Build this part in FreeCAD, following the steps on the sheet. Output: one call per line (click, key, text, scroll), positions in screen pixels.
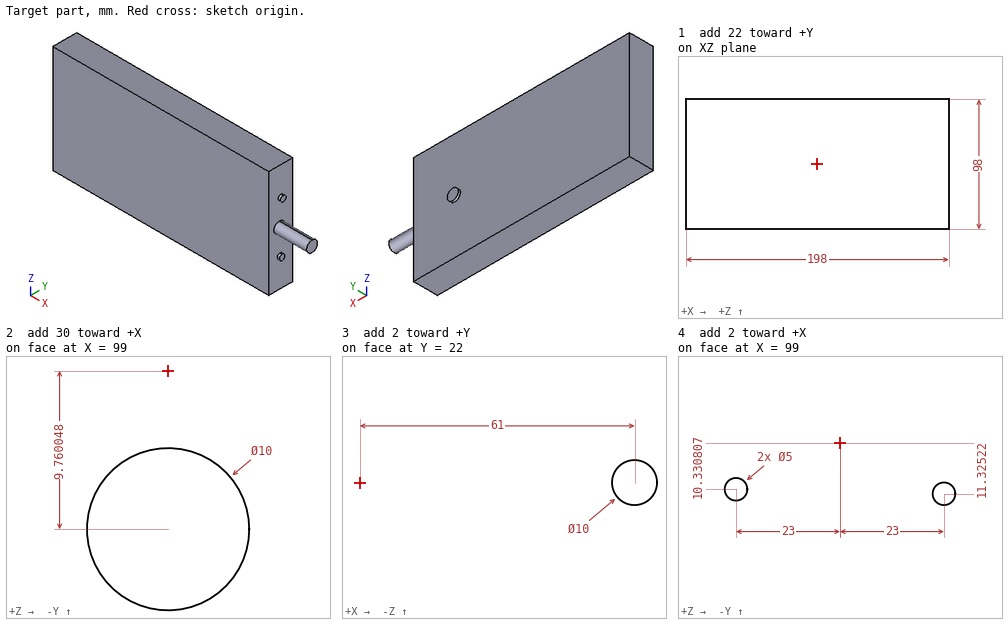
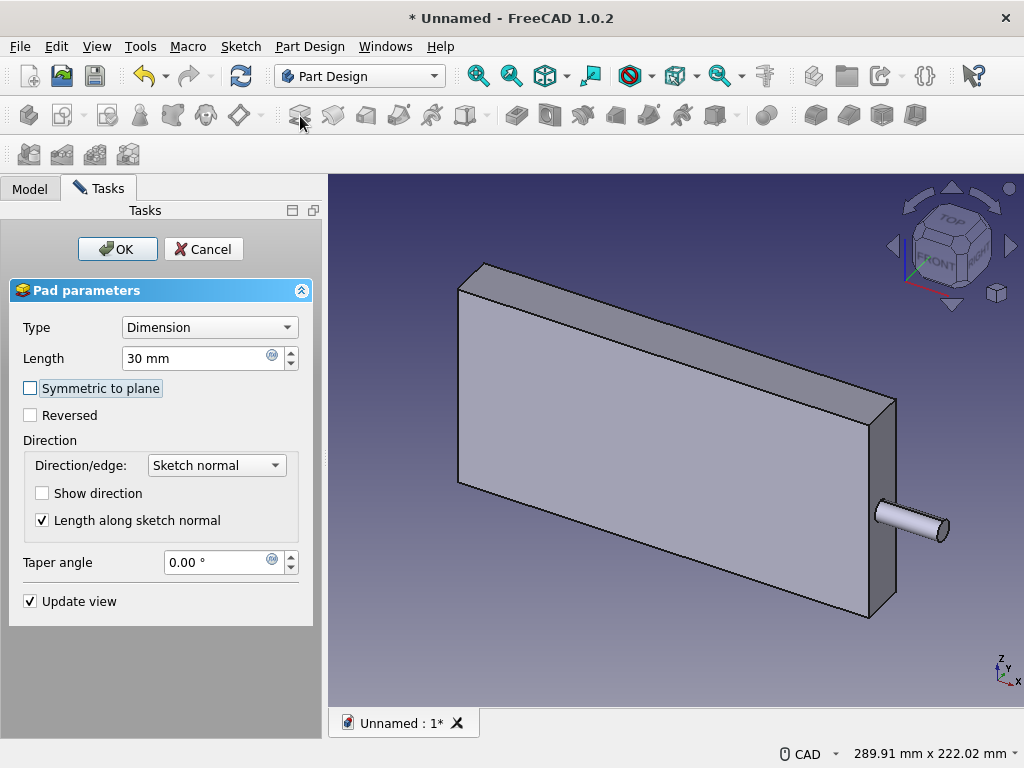
click(118, 249)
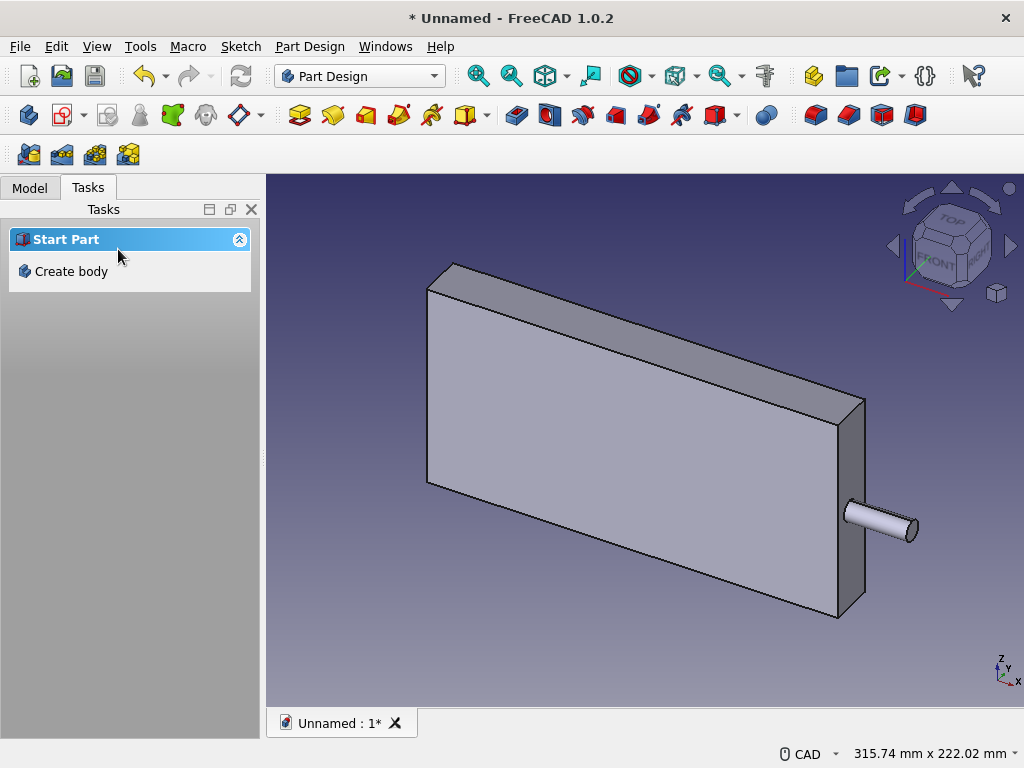
key(4)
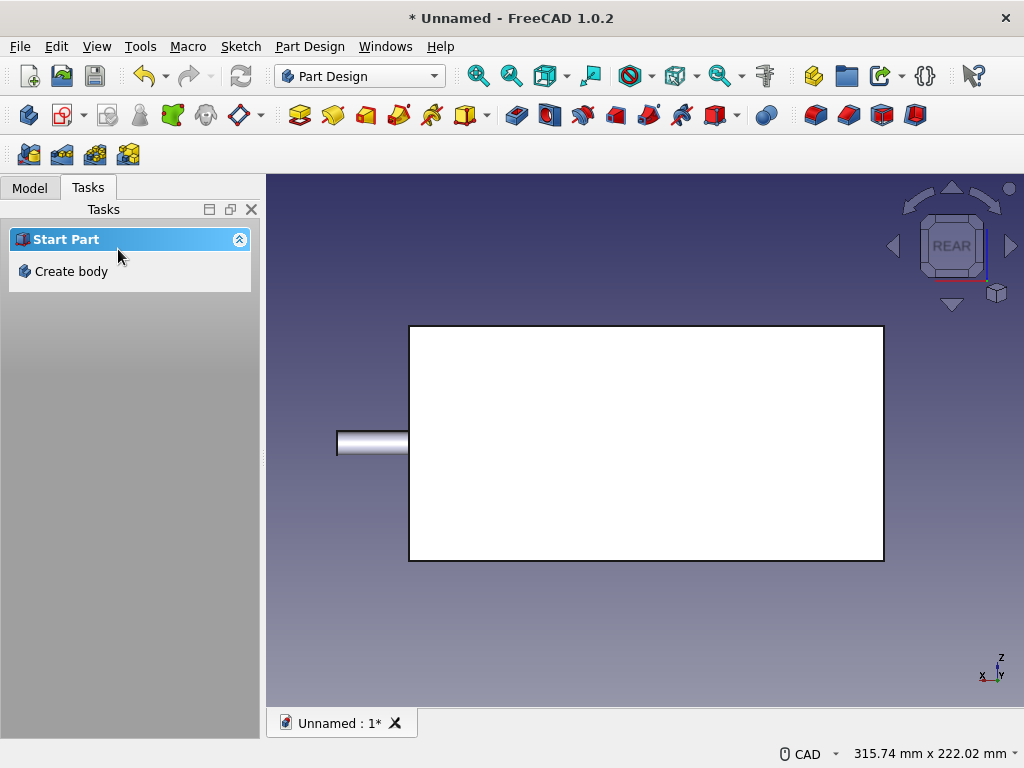
click(578, 442)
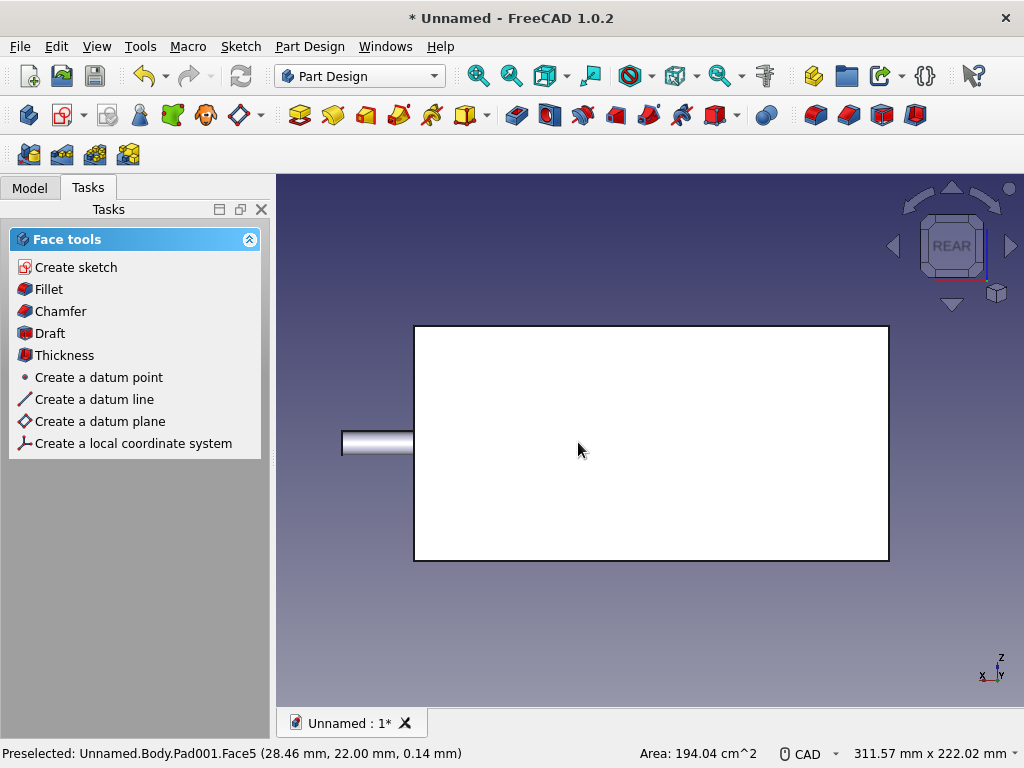
click(62, 116)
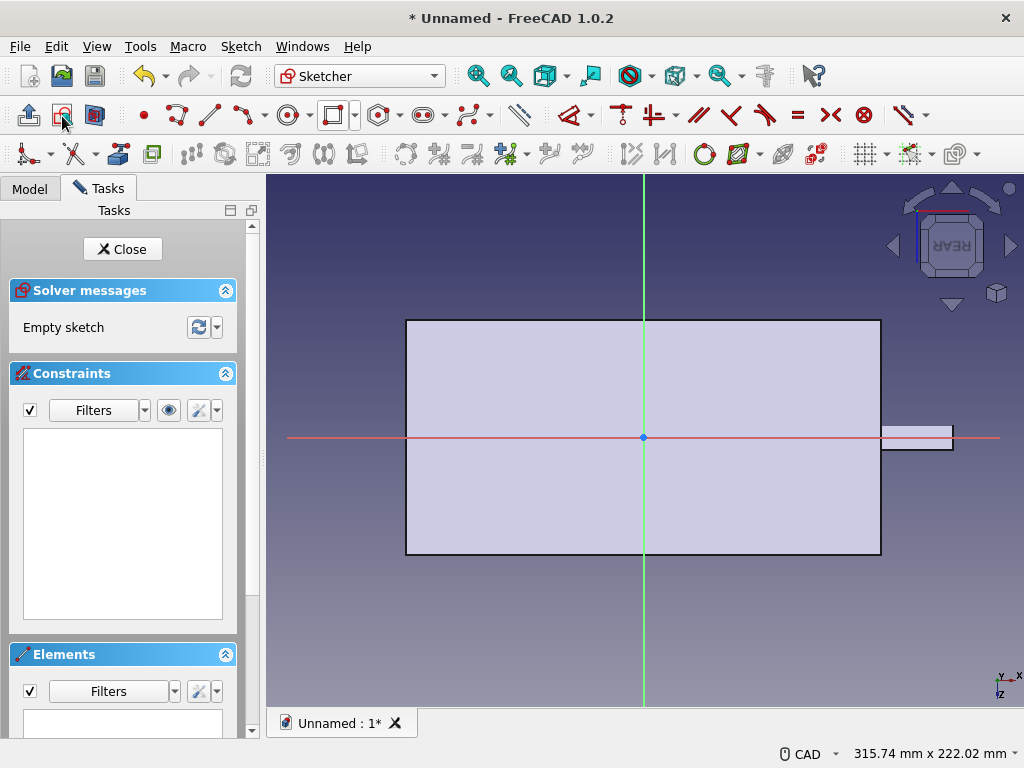
scroll(807, 437, up, 13)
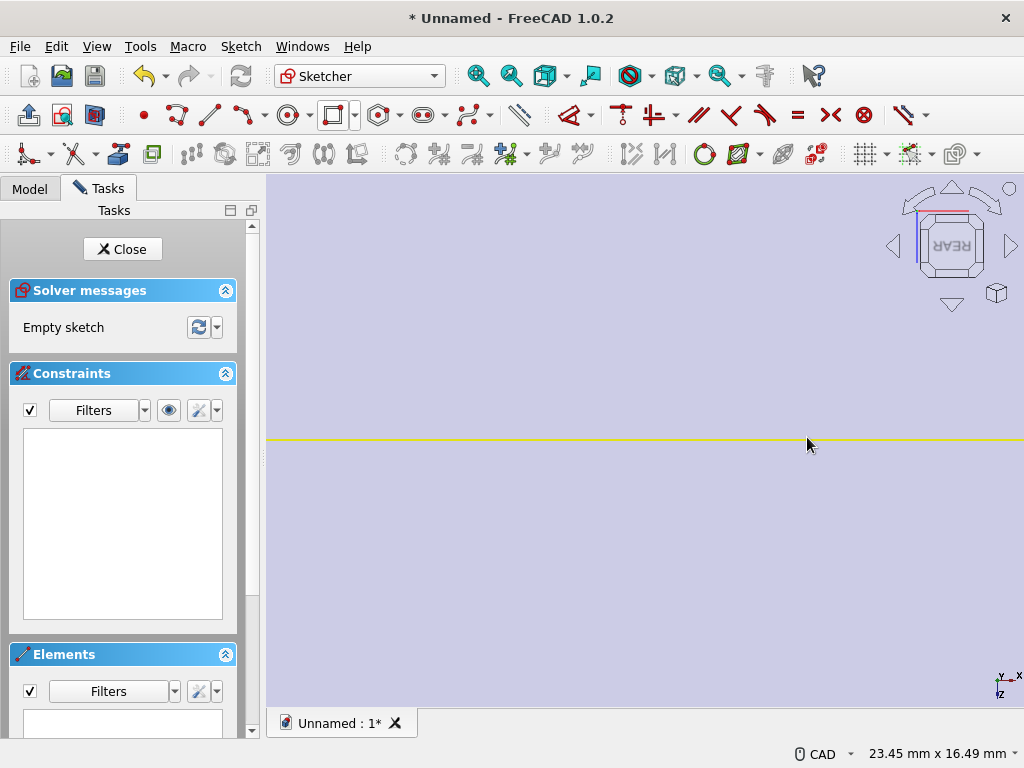
key(g)
key(c)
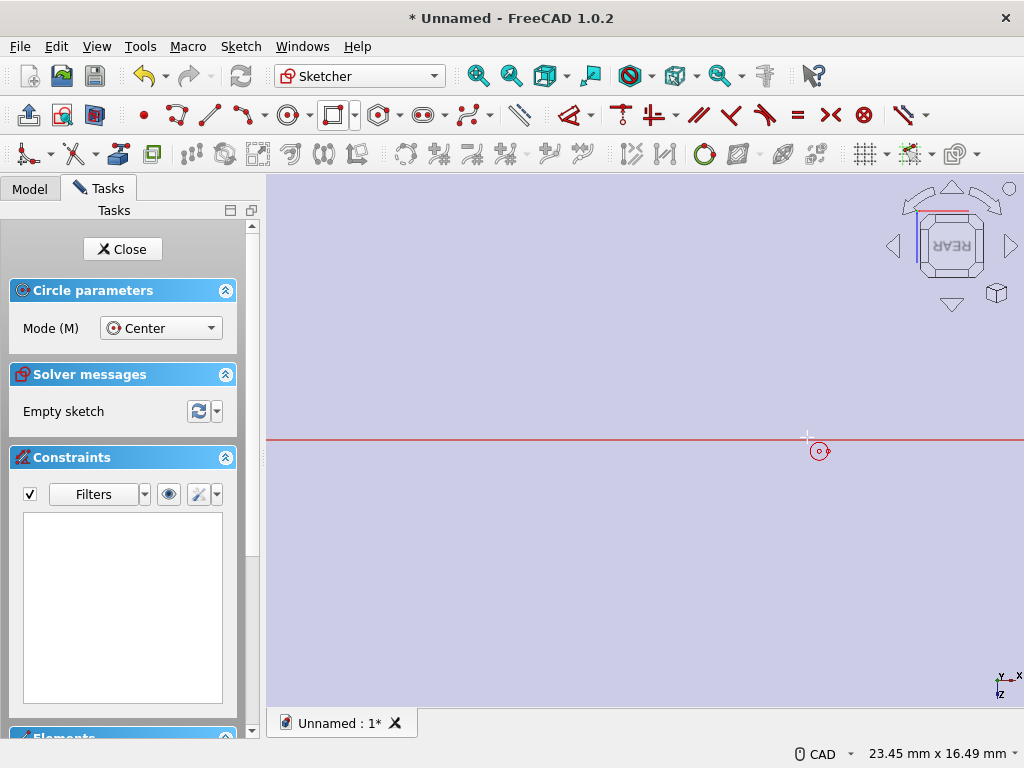
click(571, 440)
move(685, 325)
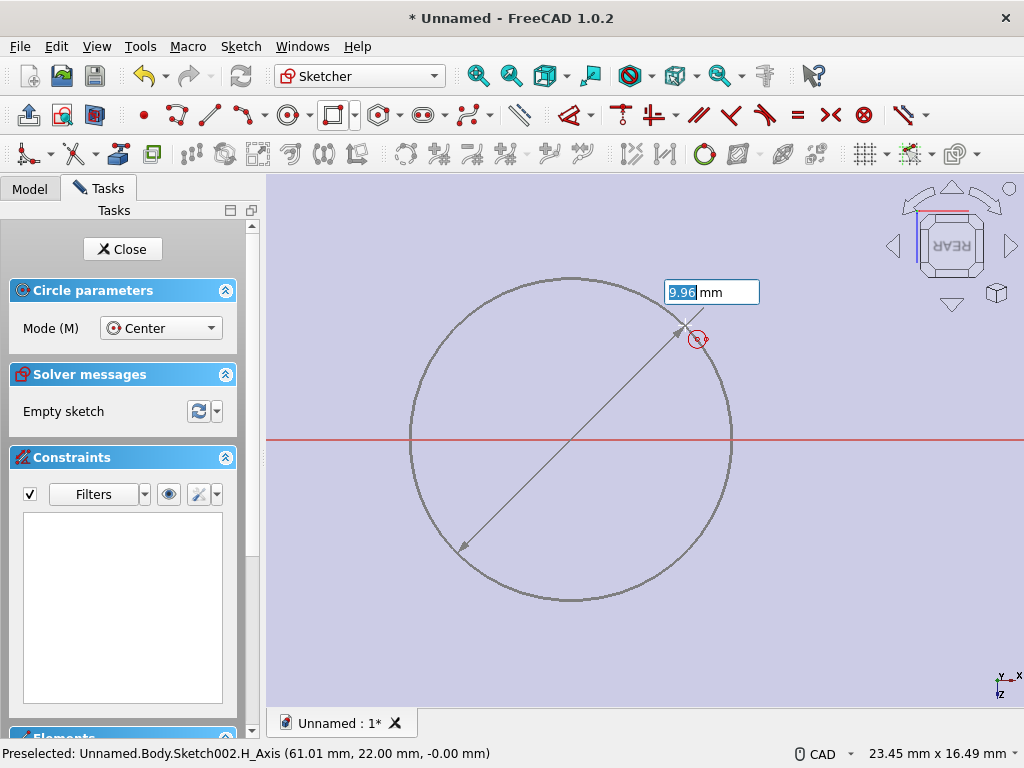
text(10)
key(Return)
key(Escape)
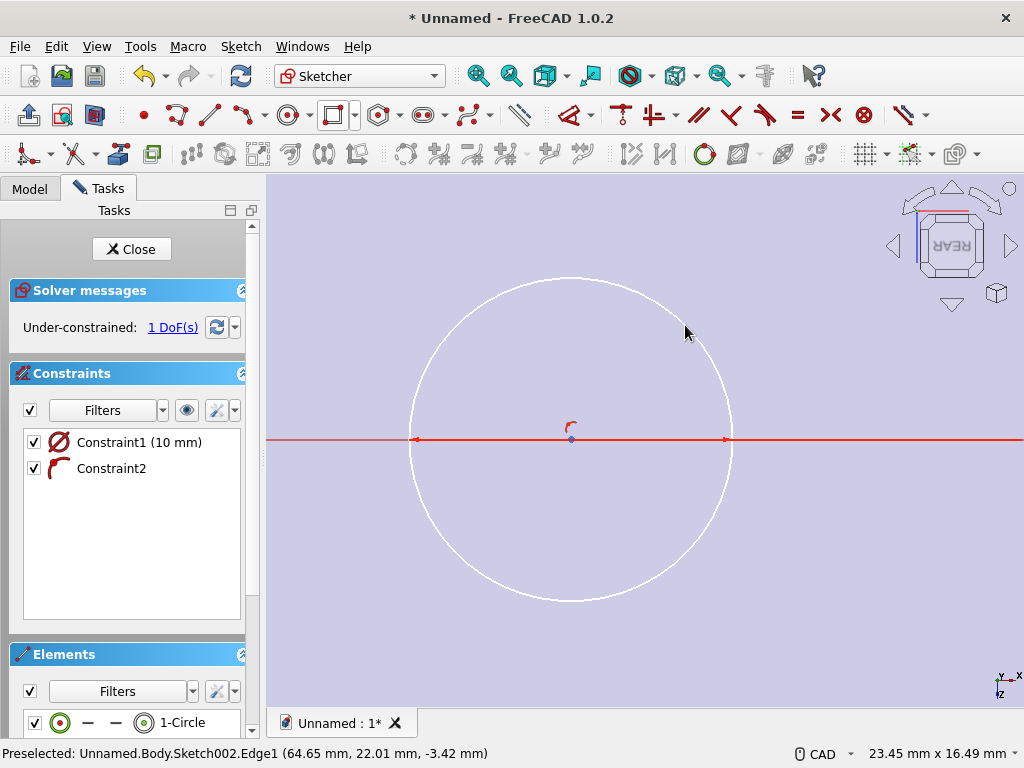
key(d)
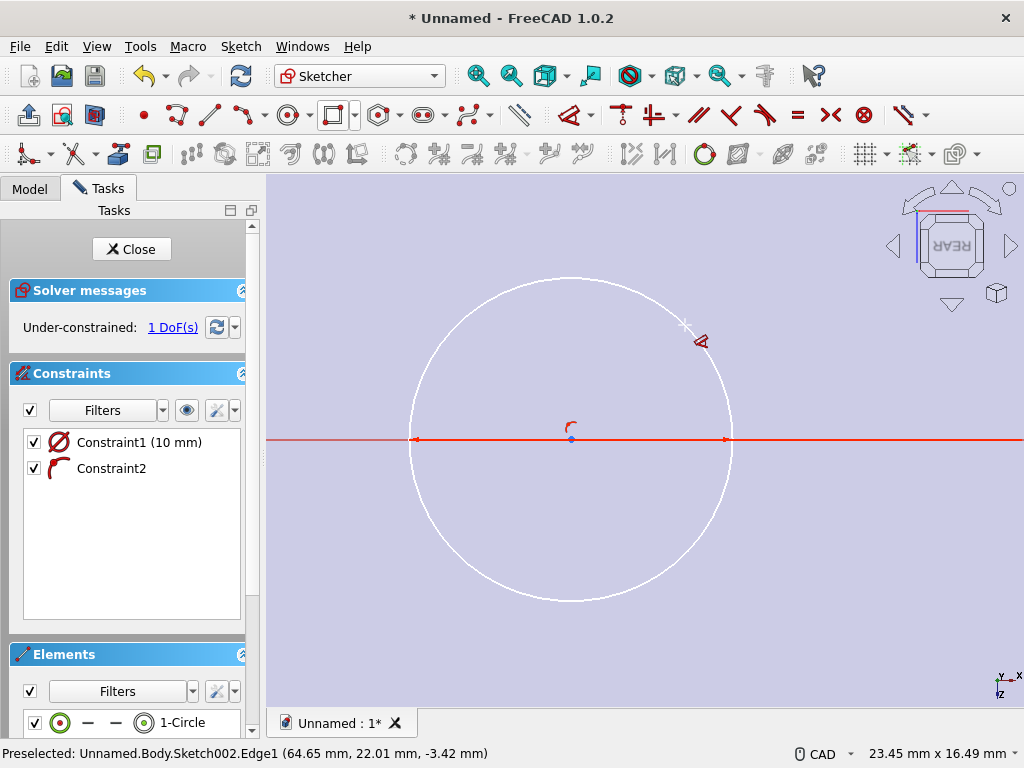
click(571, 440)
click(433, 474)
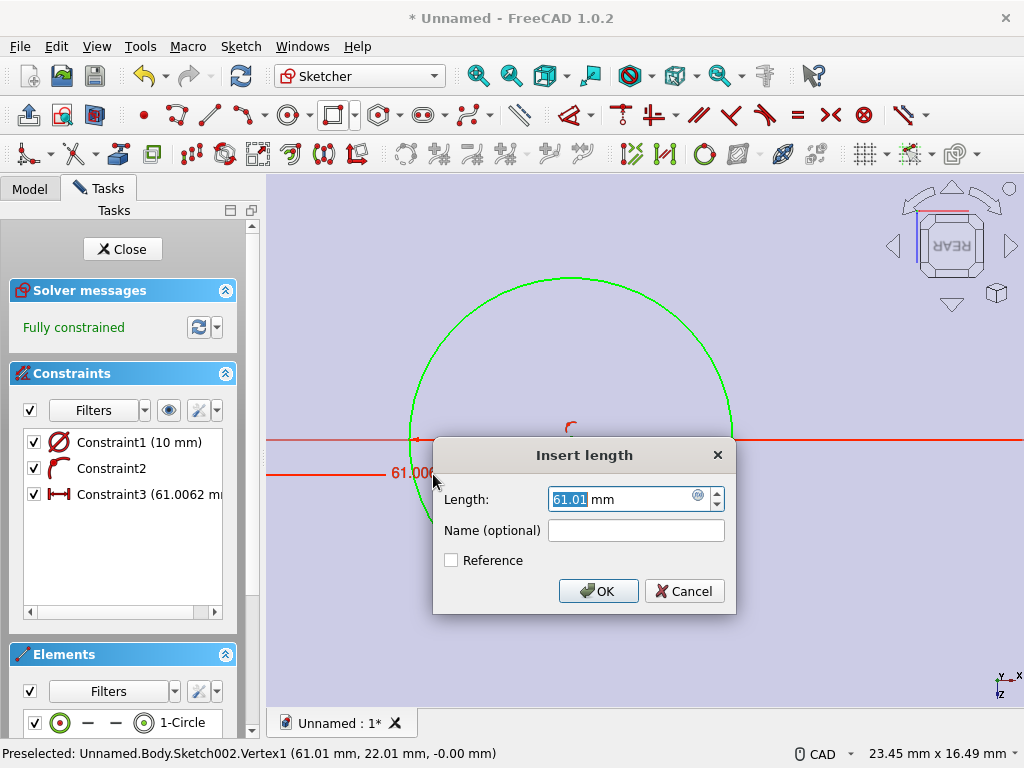
text(61)
key(Return)
key(Escape)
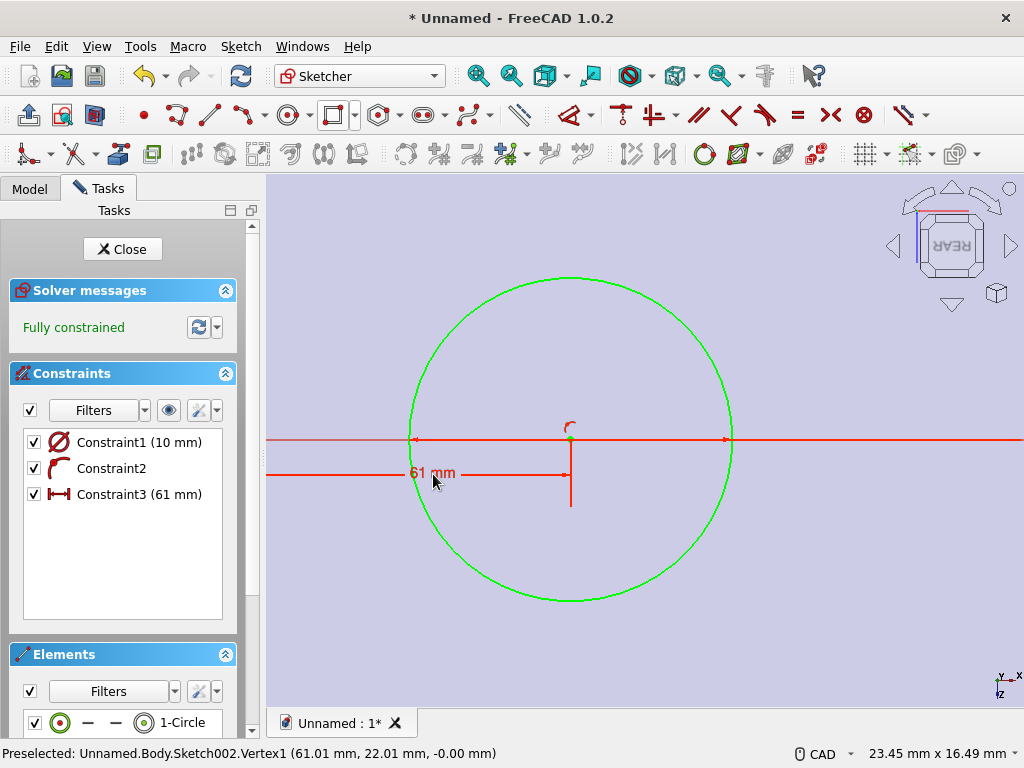
click(123, 249)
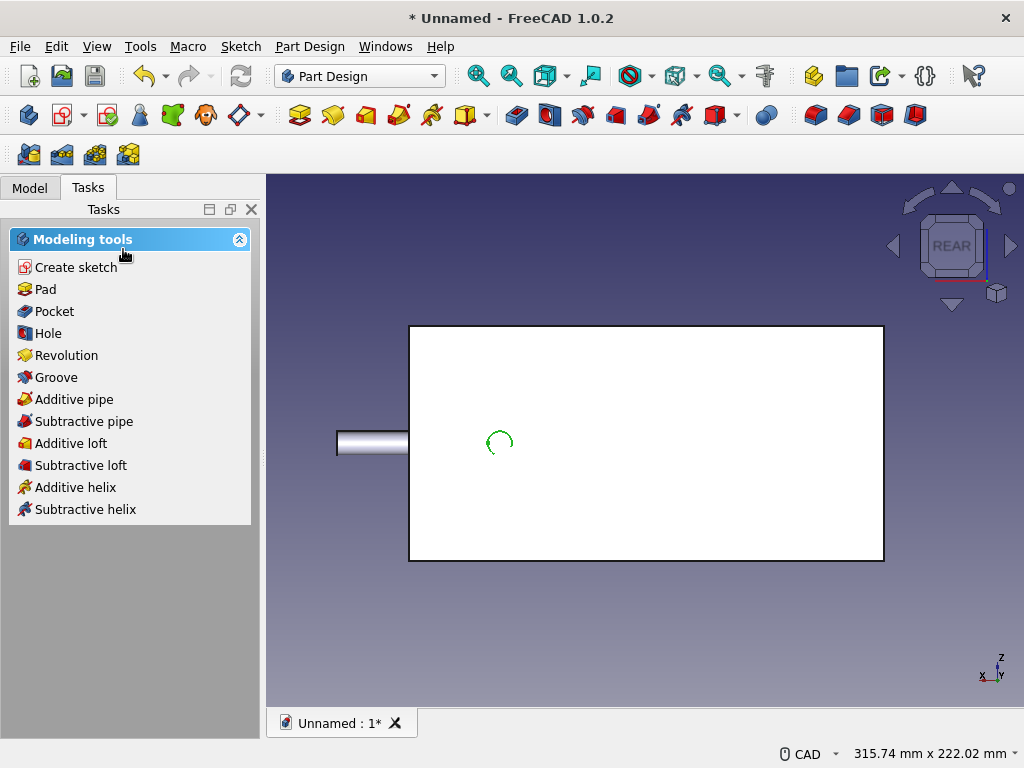
click(300, 116)